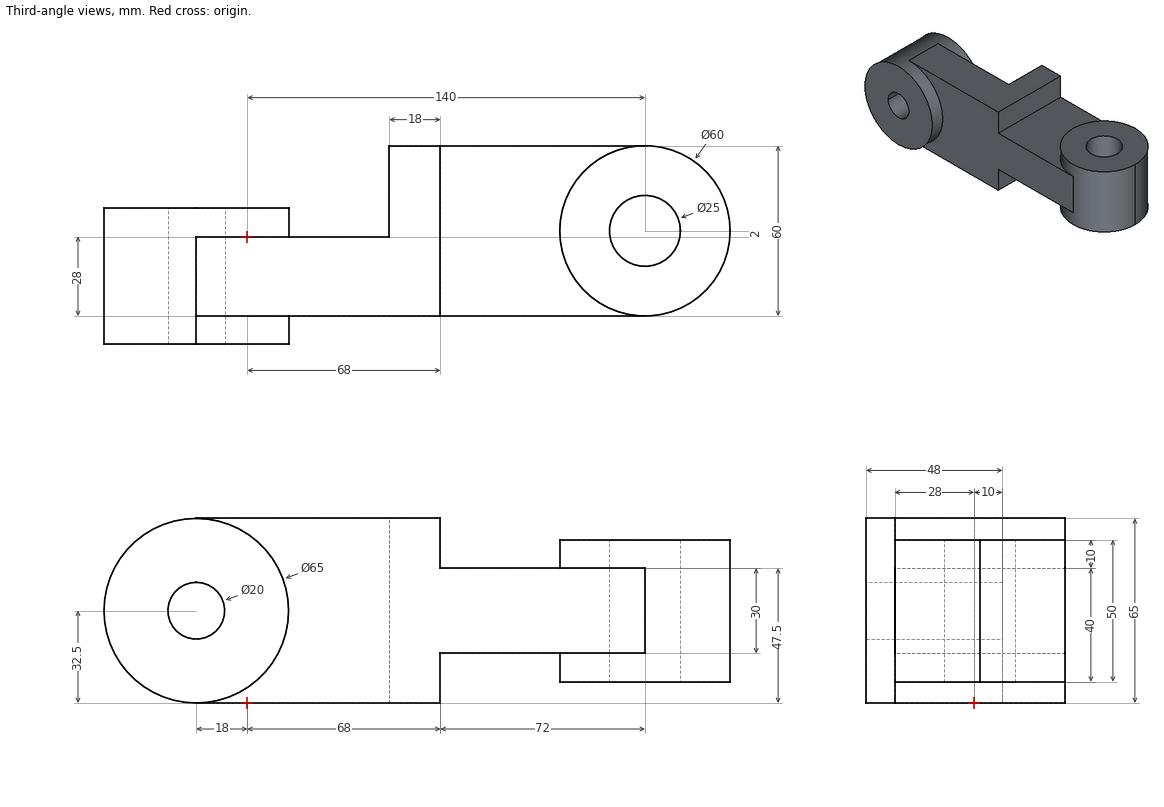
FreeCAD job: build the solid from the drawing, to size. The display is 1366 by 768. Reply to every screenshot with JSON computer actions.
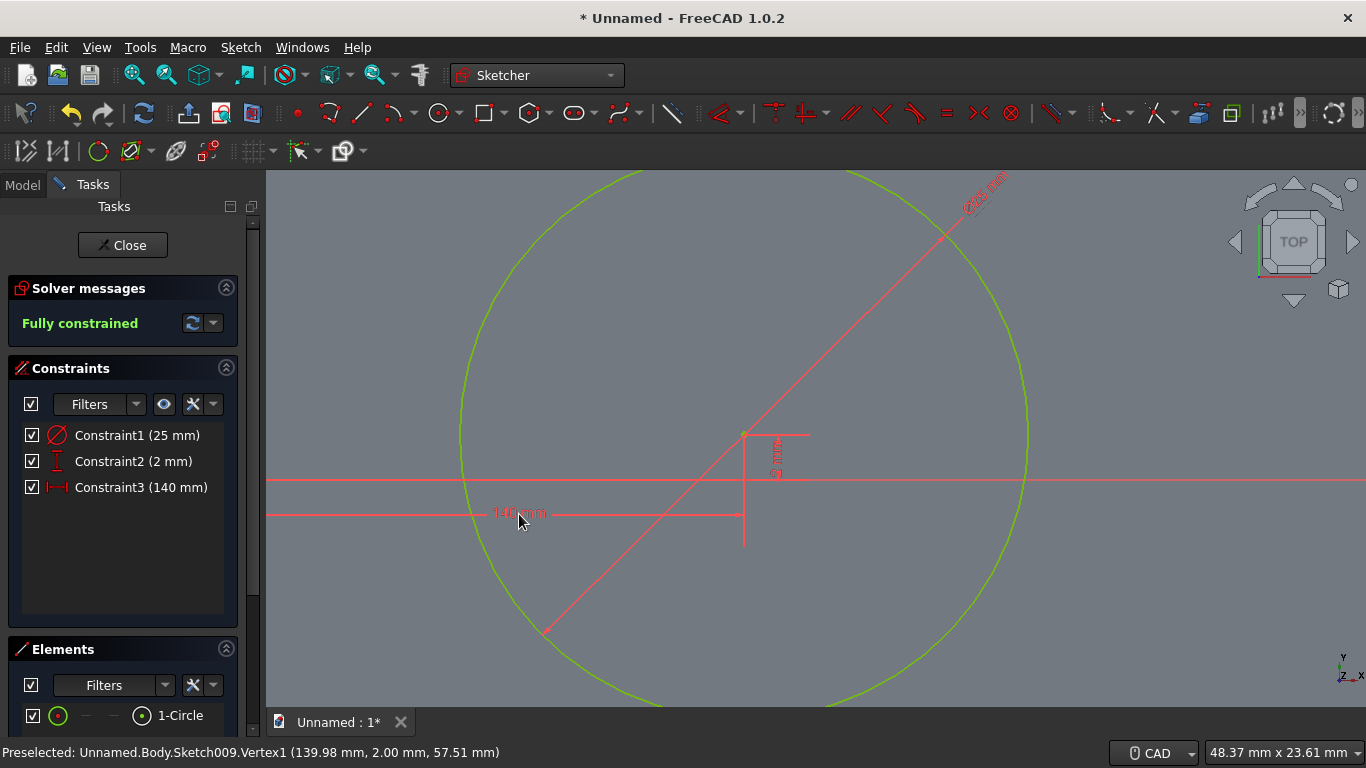
{"action": "left_click", "coordinate": [123, 245]}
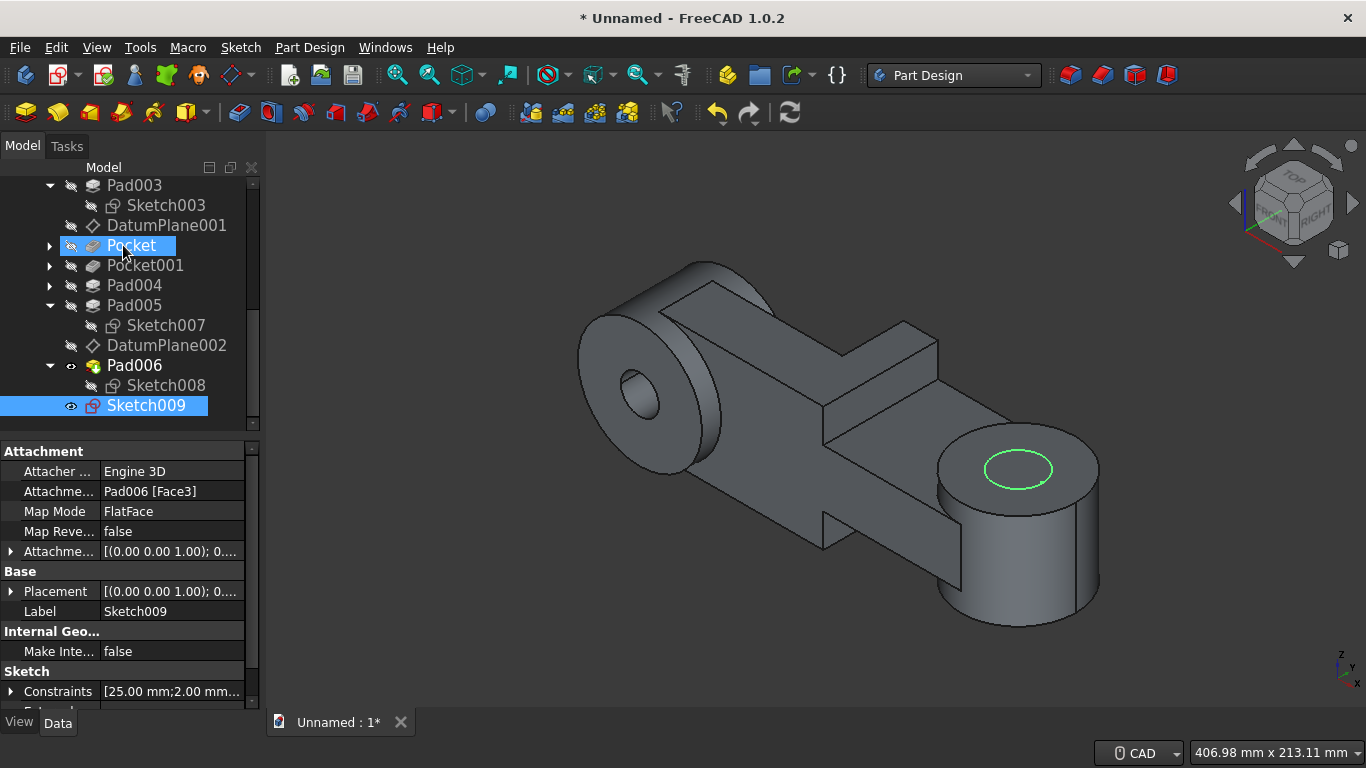
{"action": "left_click", "coordinate": [240, 112]}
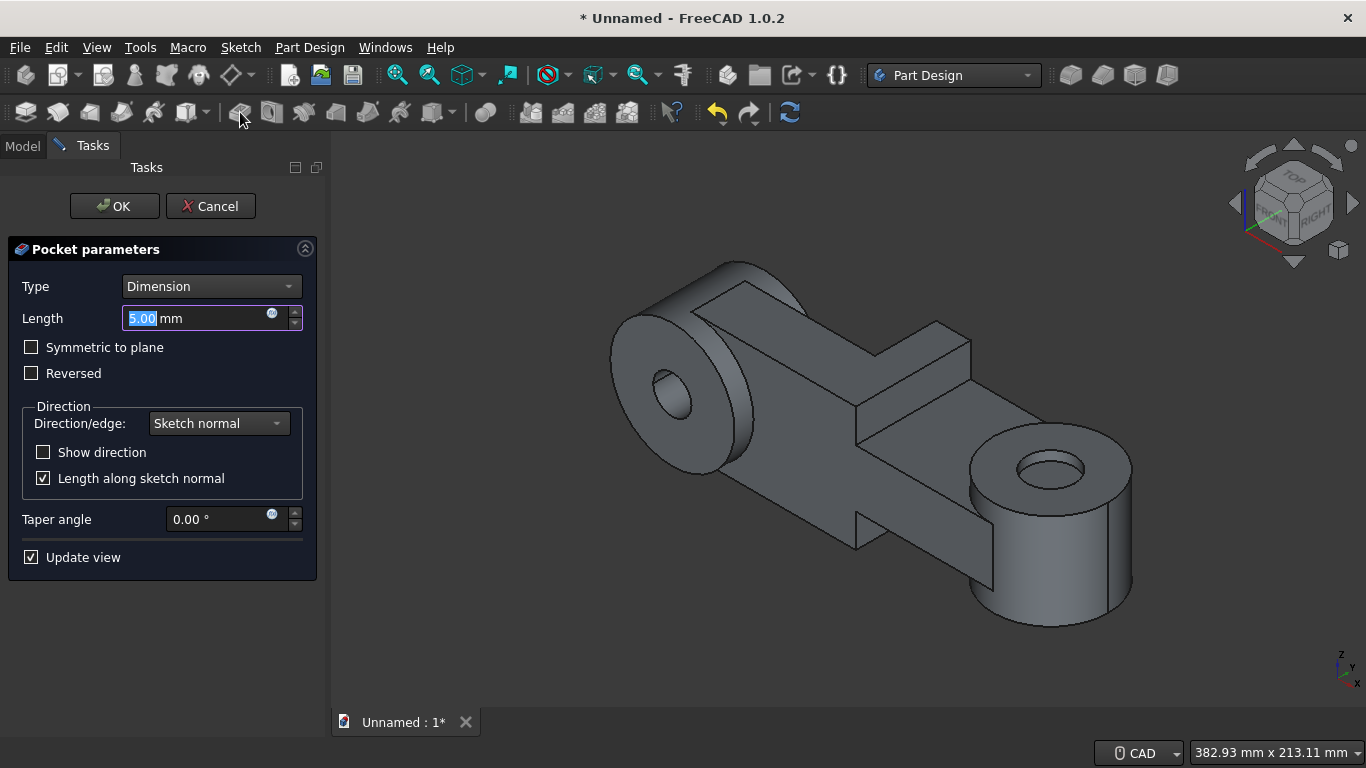
{"action": "type", "text": "50"}
{"action": "key", "text": "Tab"}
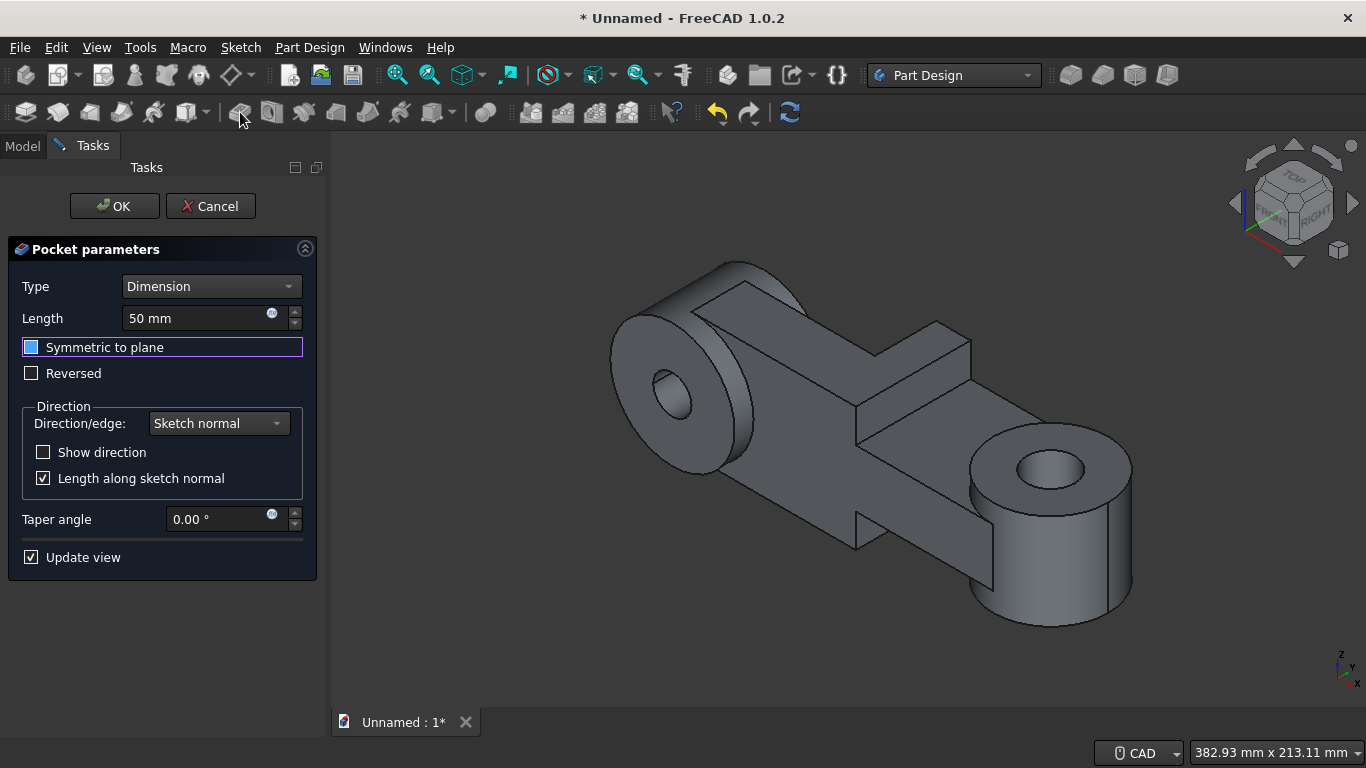
{"action": "left_click", "coordinate": [115, 206]}